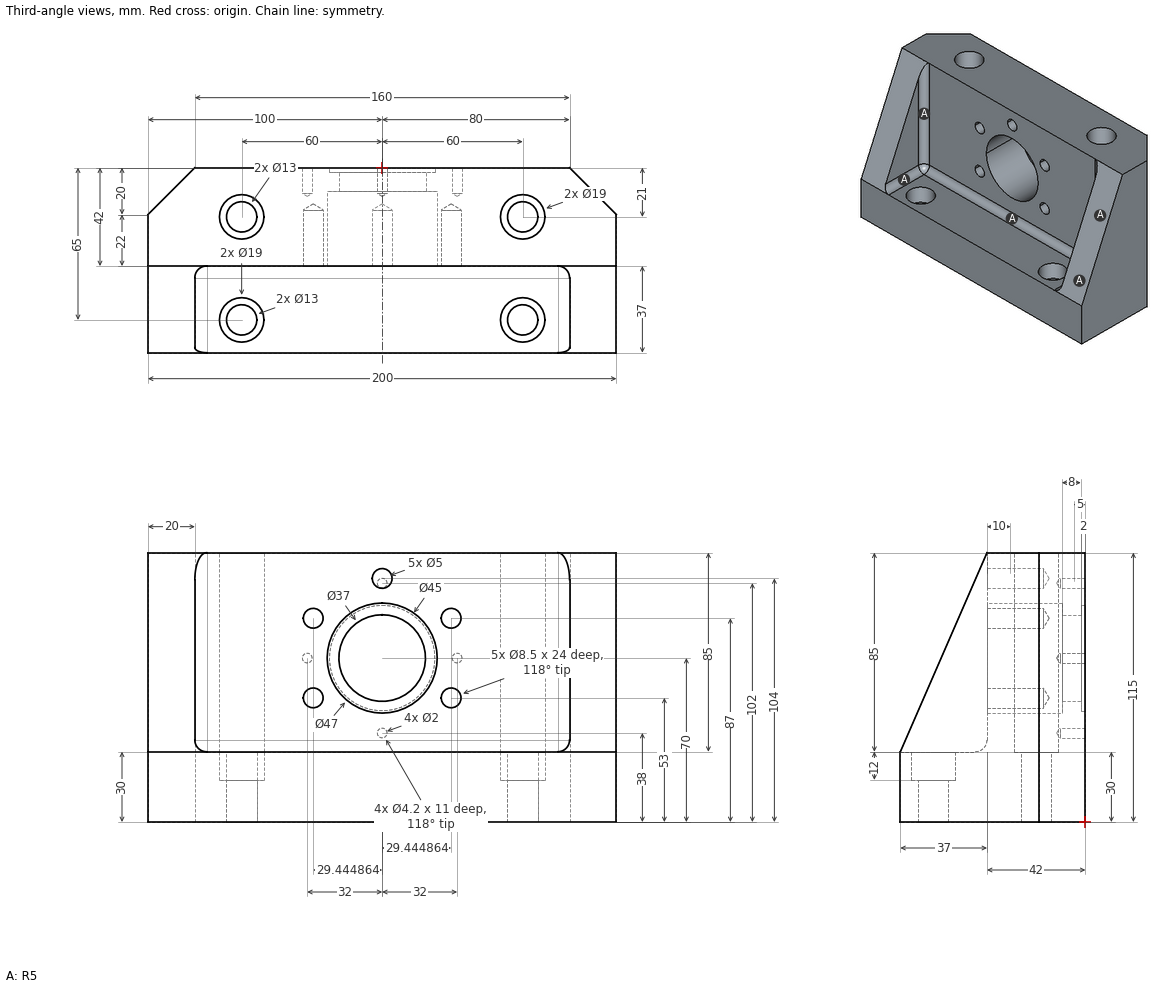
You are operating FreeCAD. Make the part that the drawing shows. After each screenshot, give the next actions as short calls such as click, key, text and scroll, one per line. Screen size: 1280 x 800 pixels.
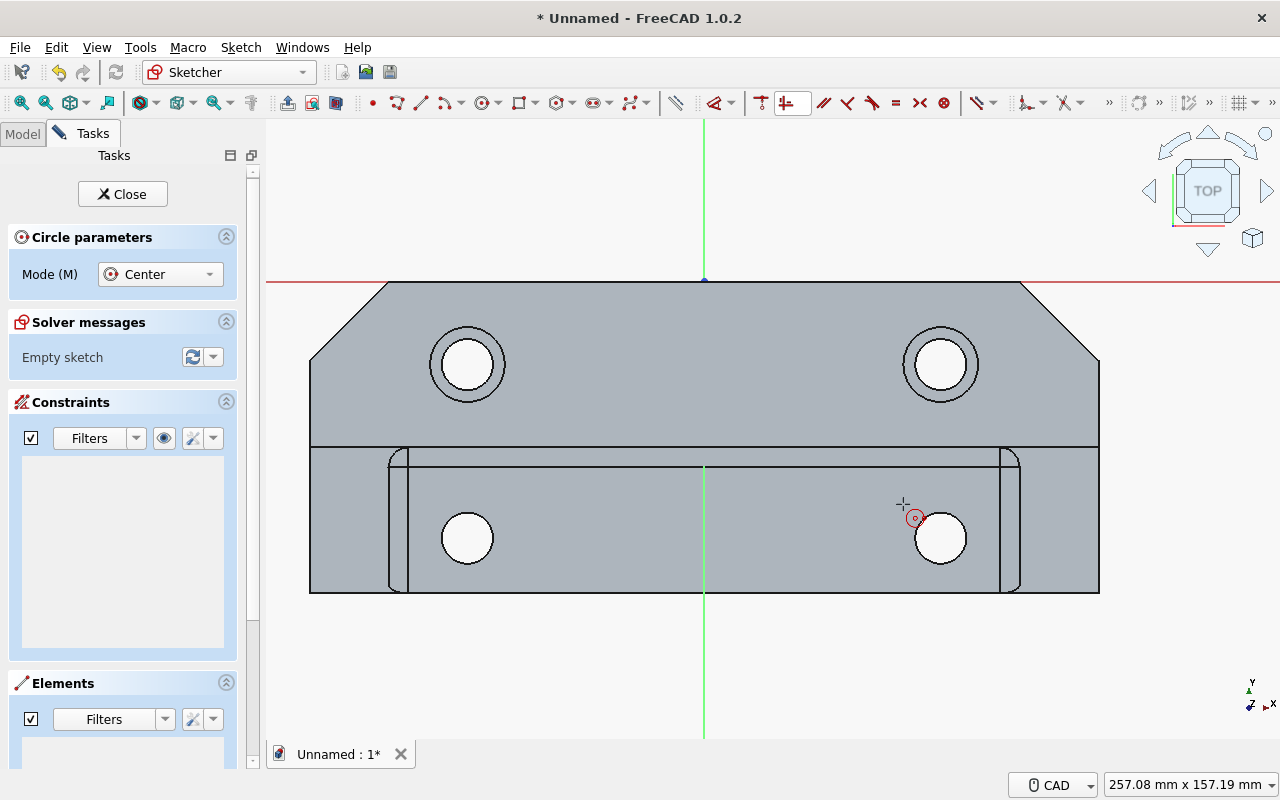
click(467, 538)
move(494, 512)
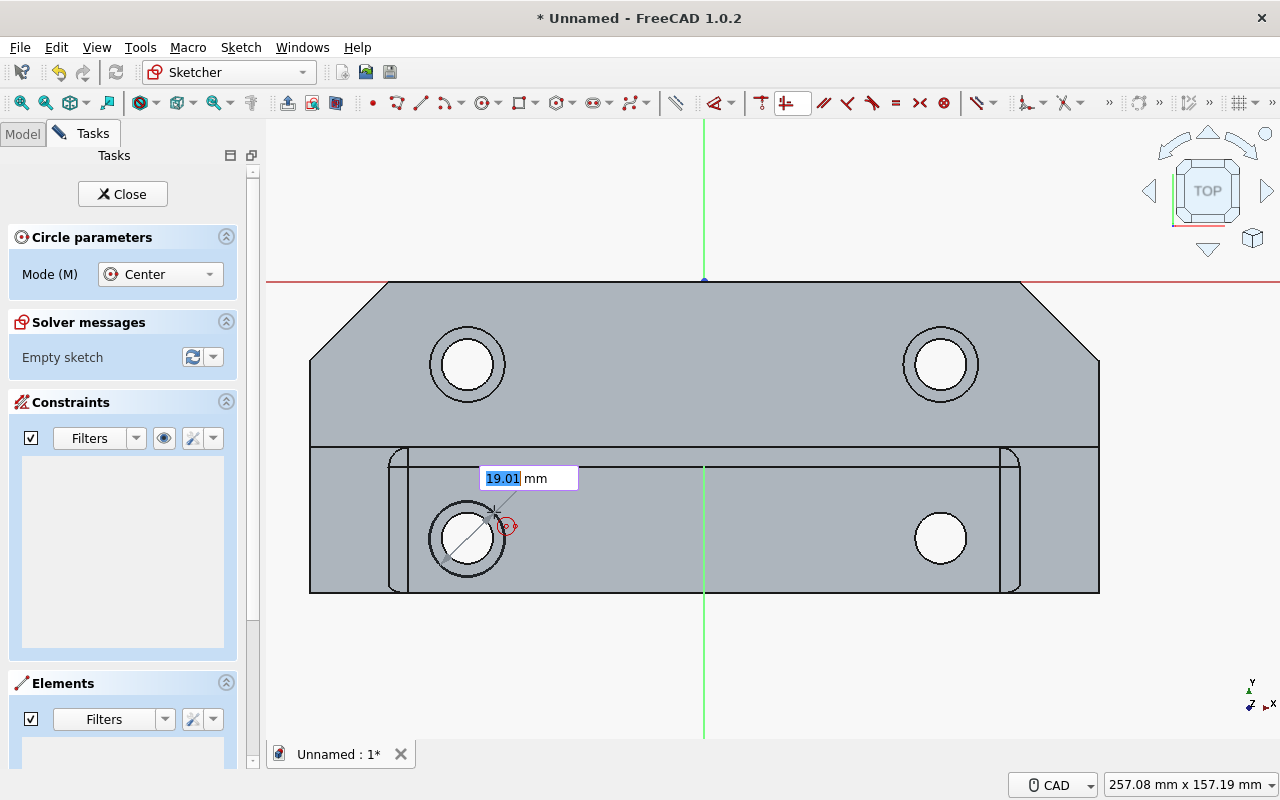
text(19)
key(Return)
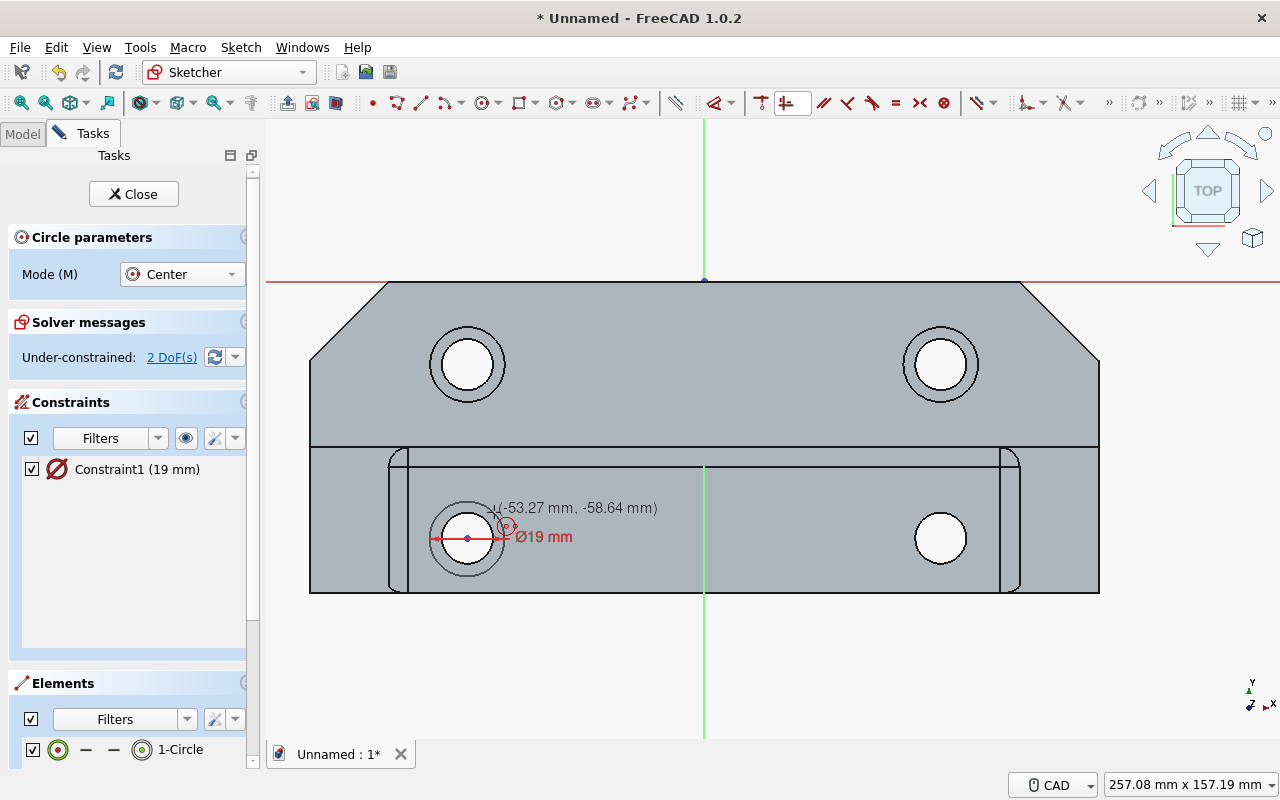
click(941, 538)
move(967, 512)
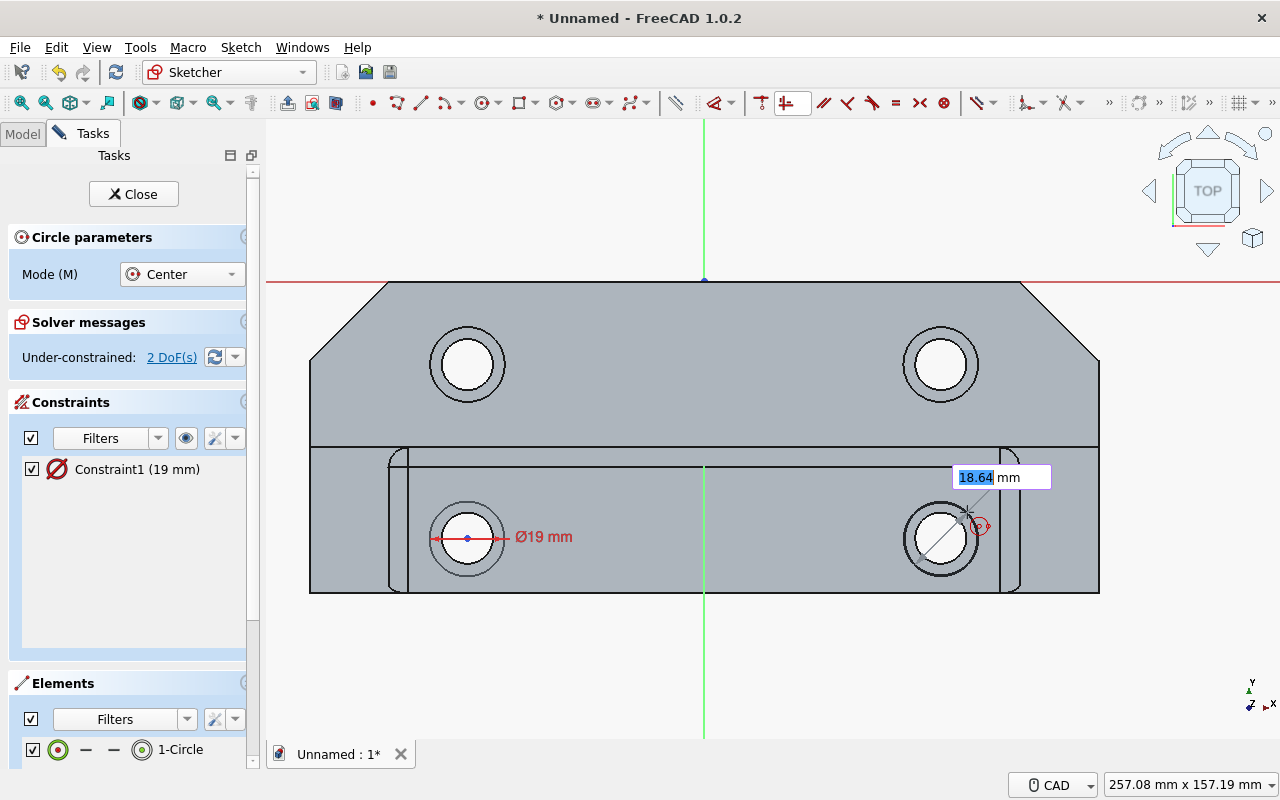
text(19)
key(Return)
key(Escape)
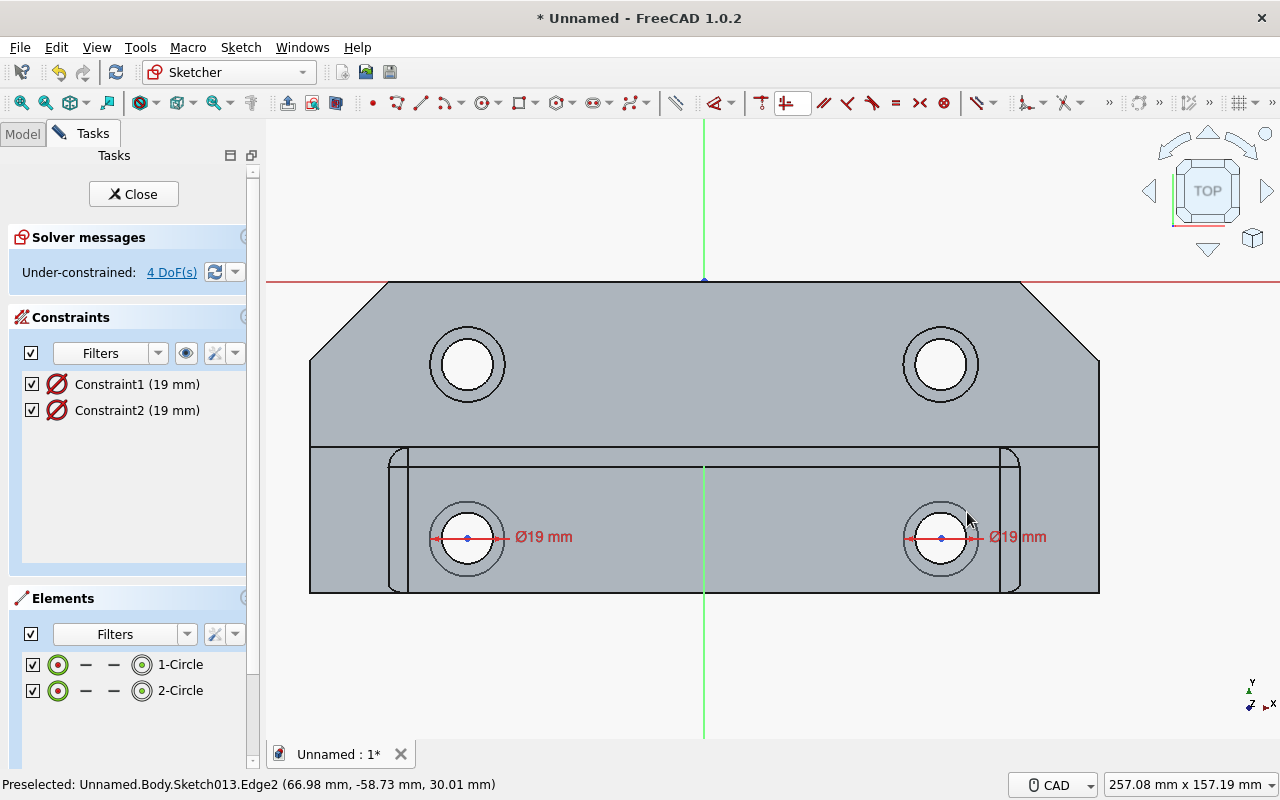
click(467, 539)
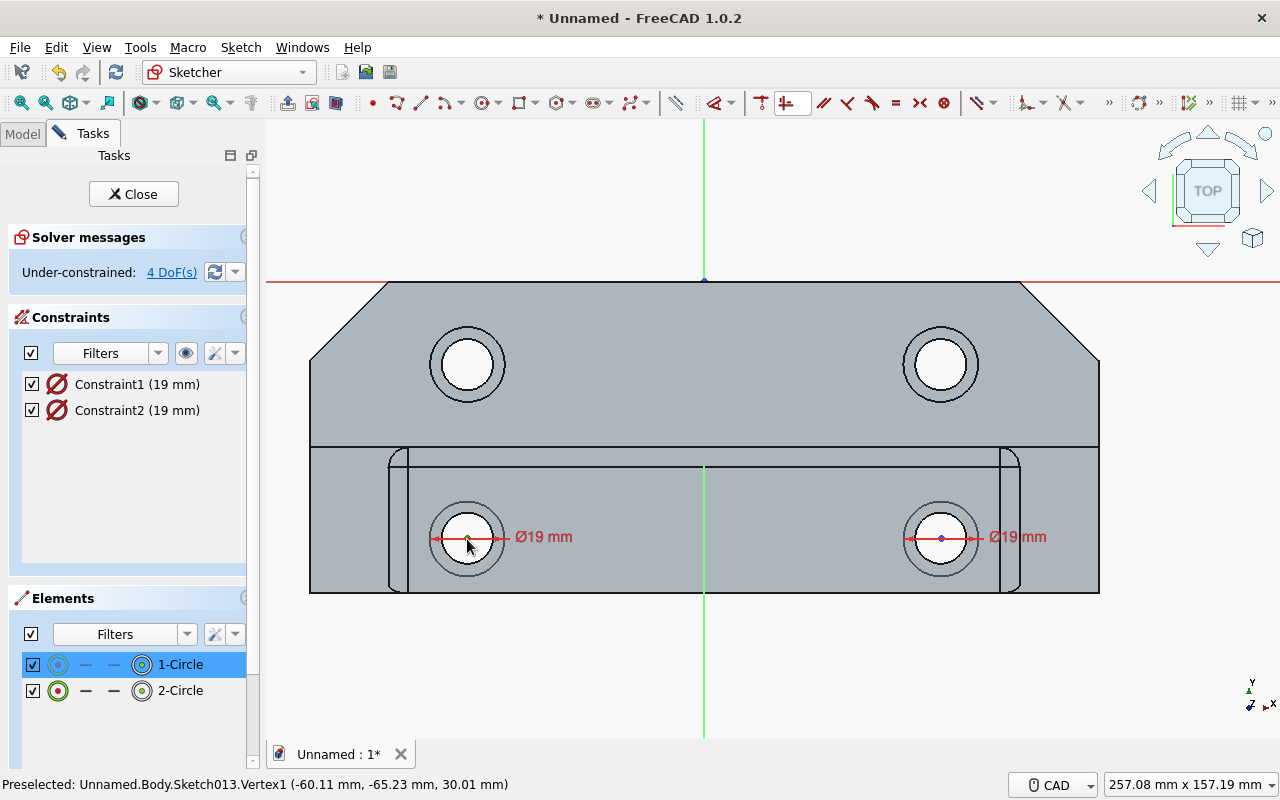
click(941, 539)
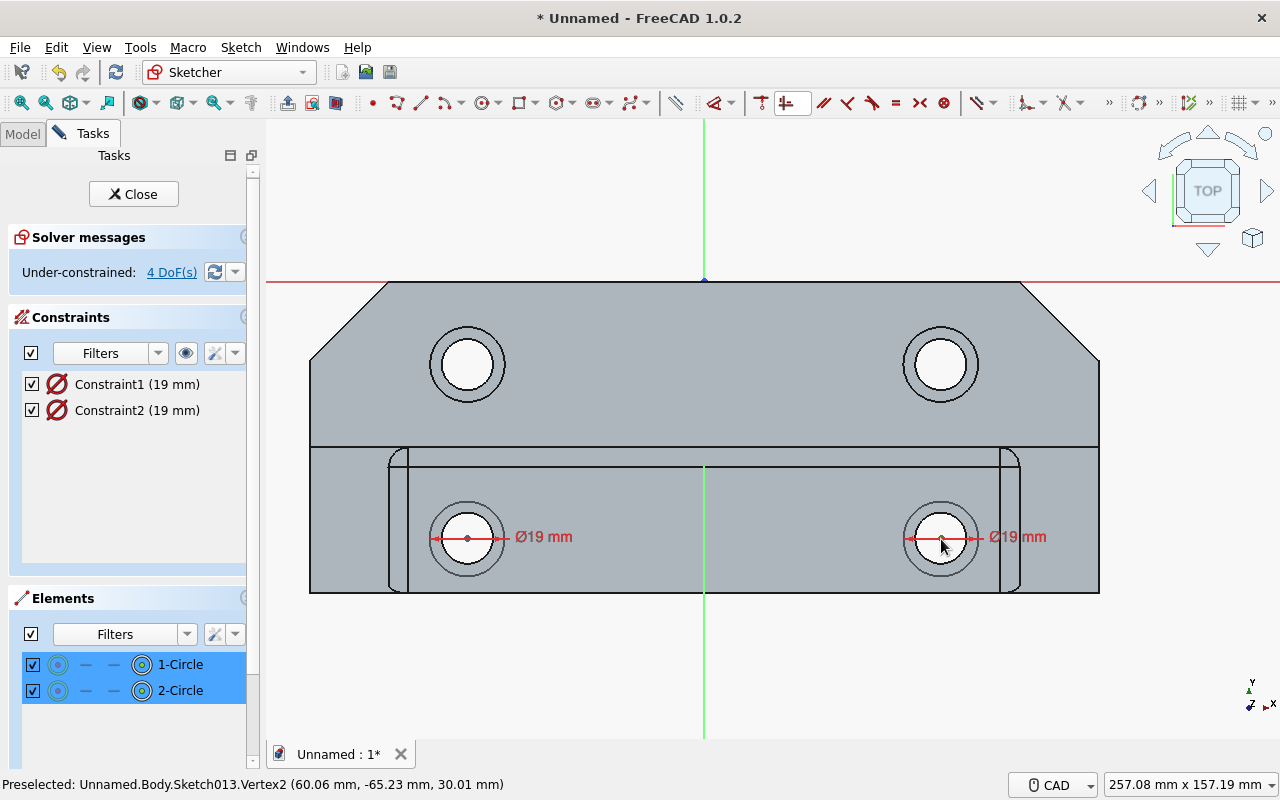
click(806, 104)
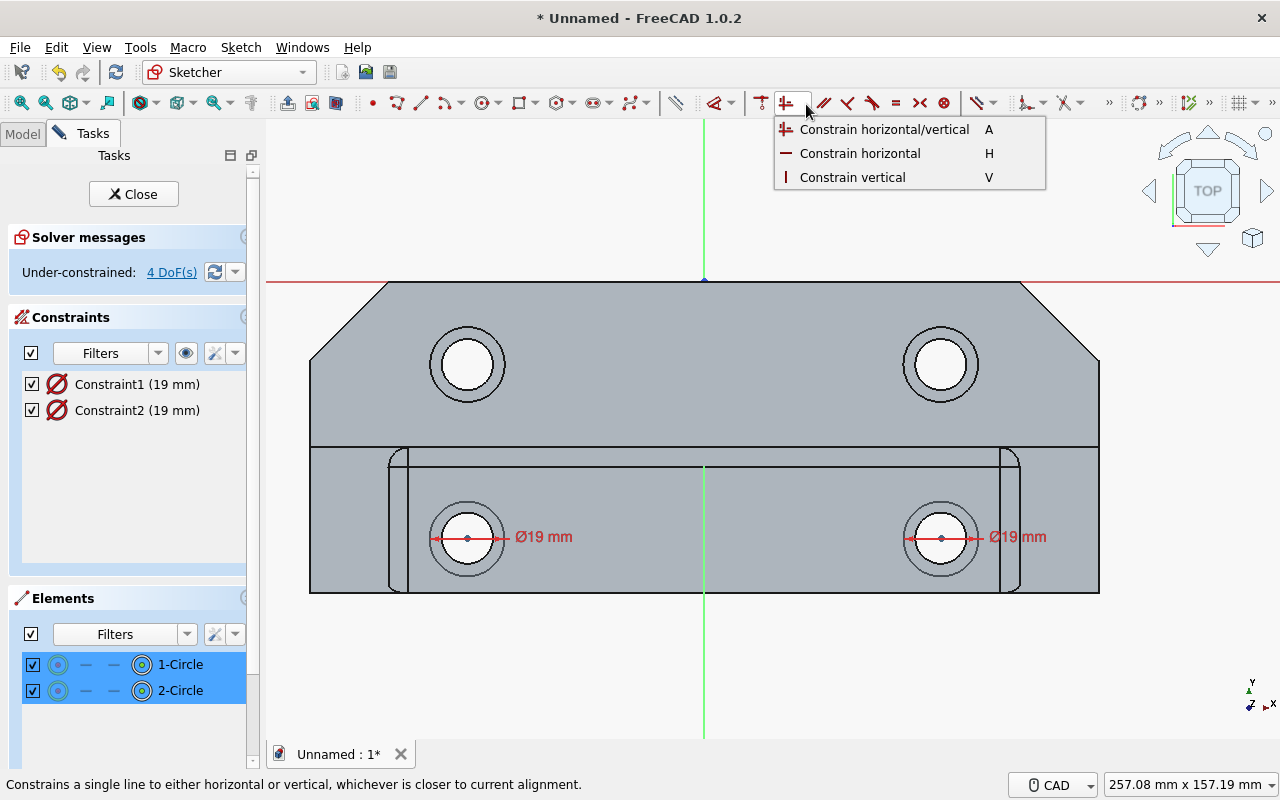
click(910, 153)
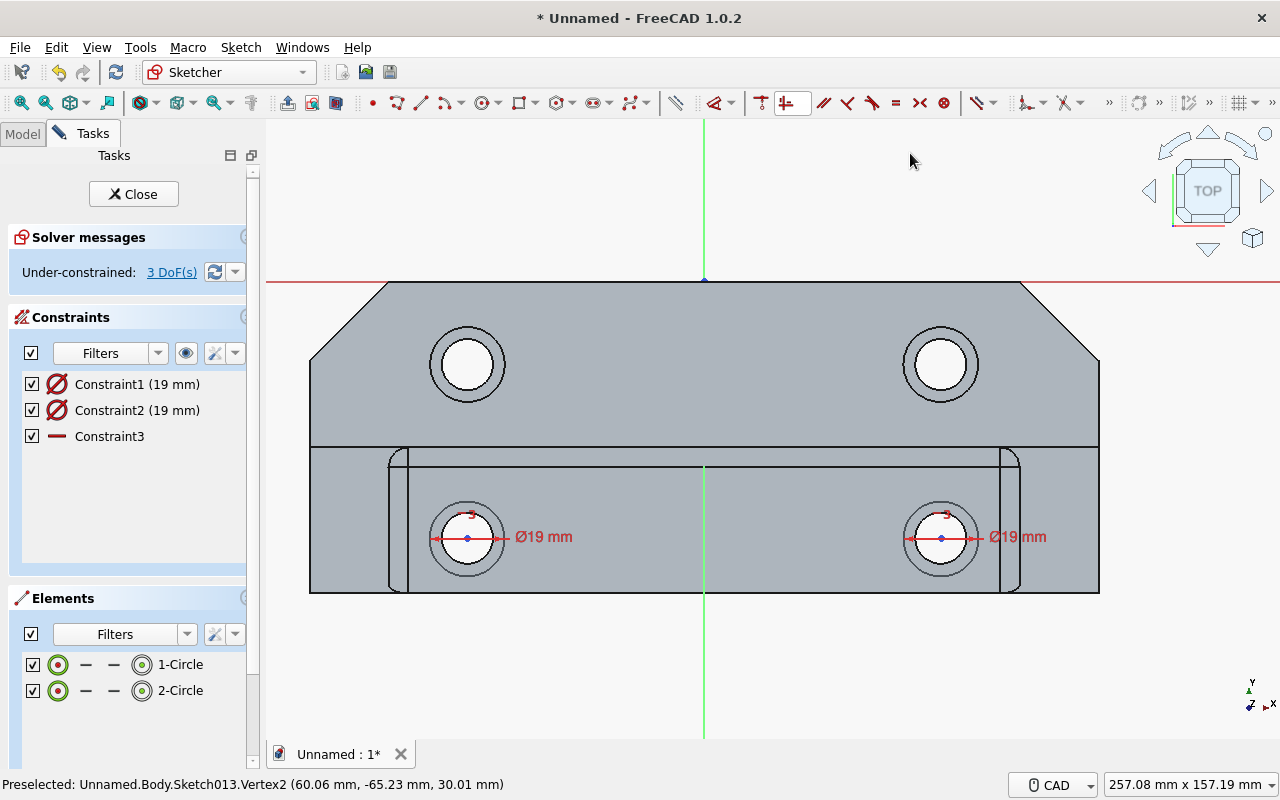
key(d)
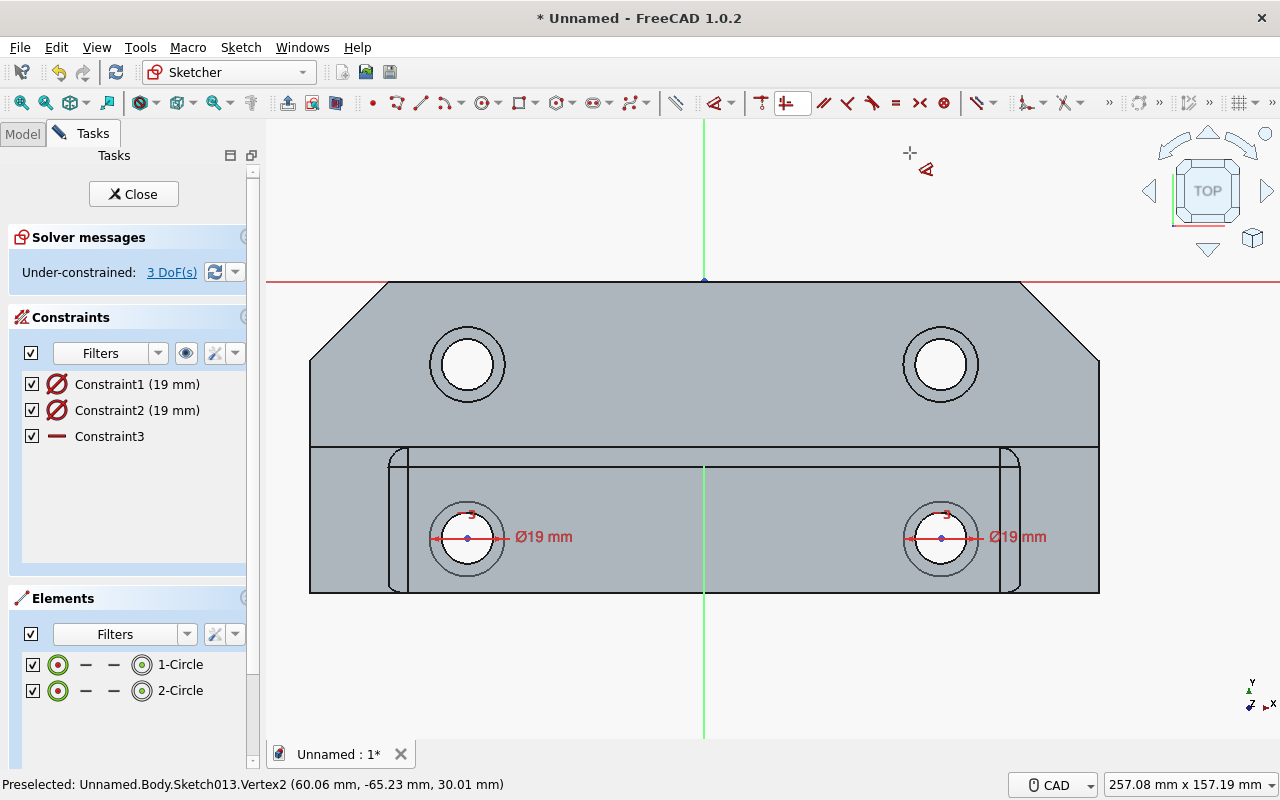
click(467, 539)
click(586, 248)